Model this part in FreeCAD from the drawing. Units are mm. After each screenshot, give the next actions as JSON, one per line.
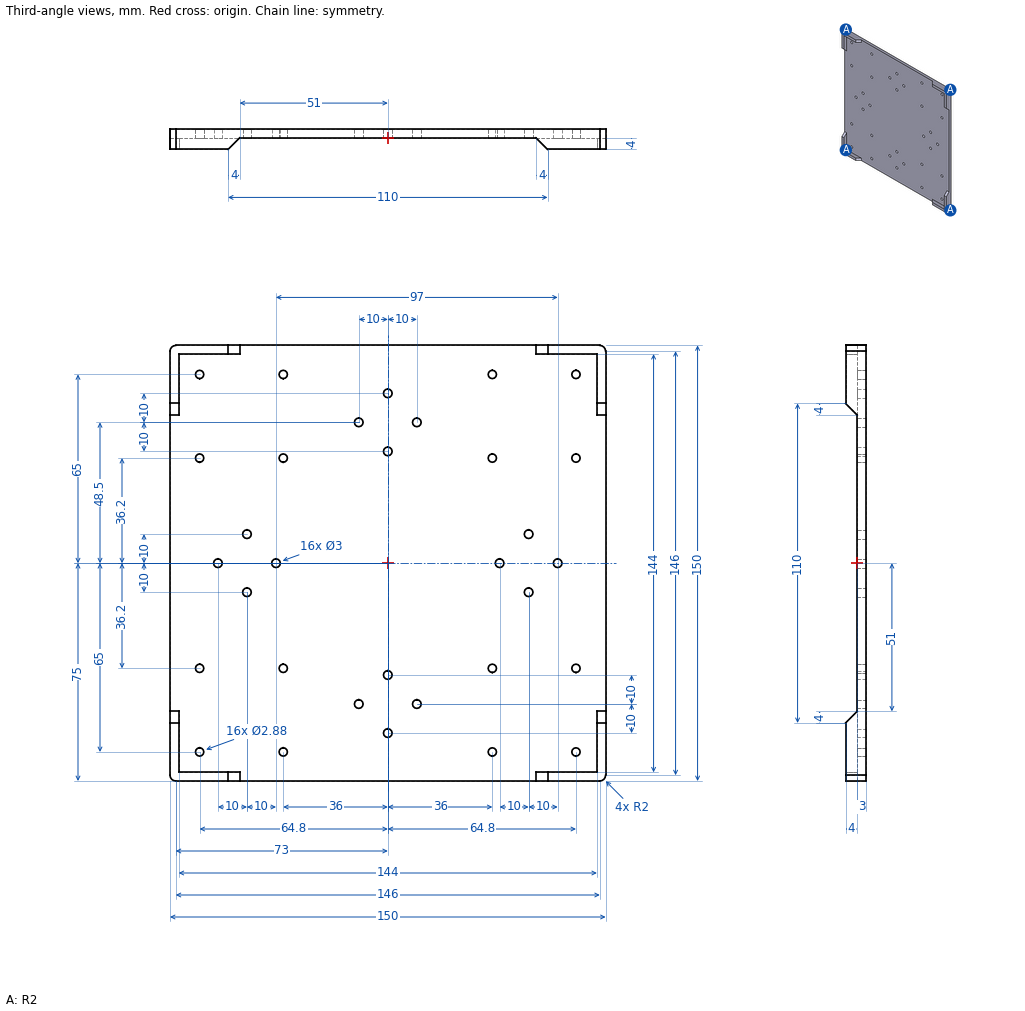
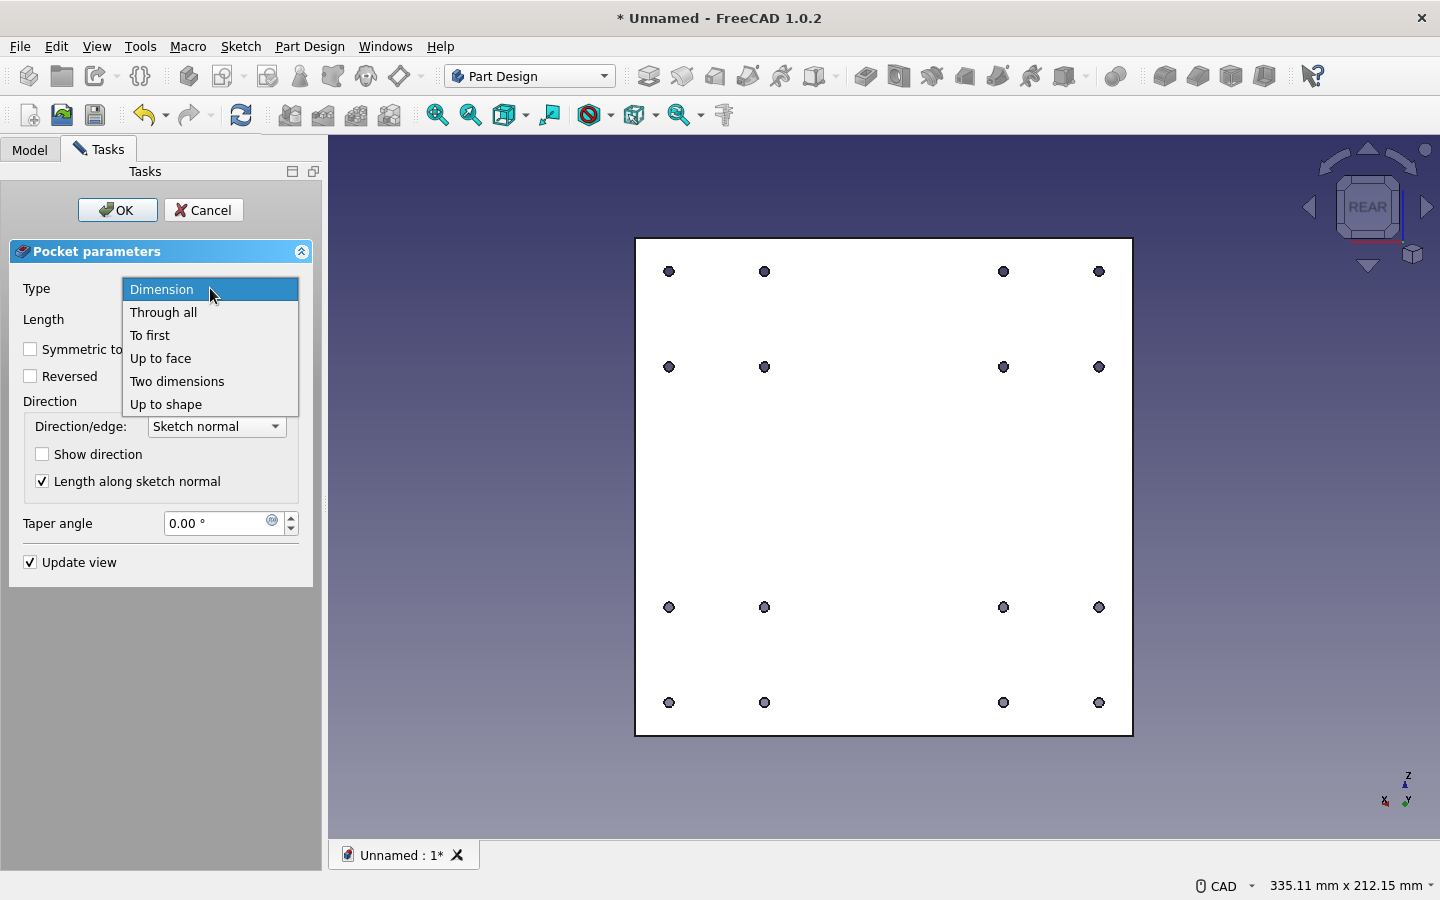
{"action": "left_click", "coordinate": [208, 312]}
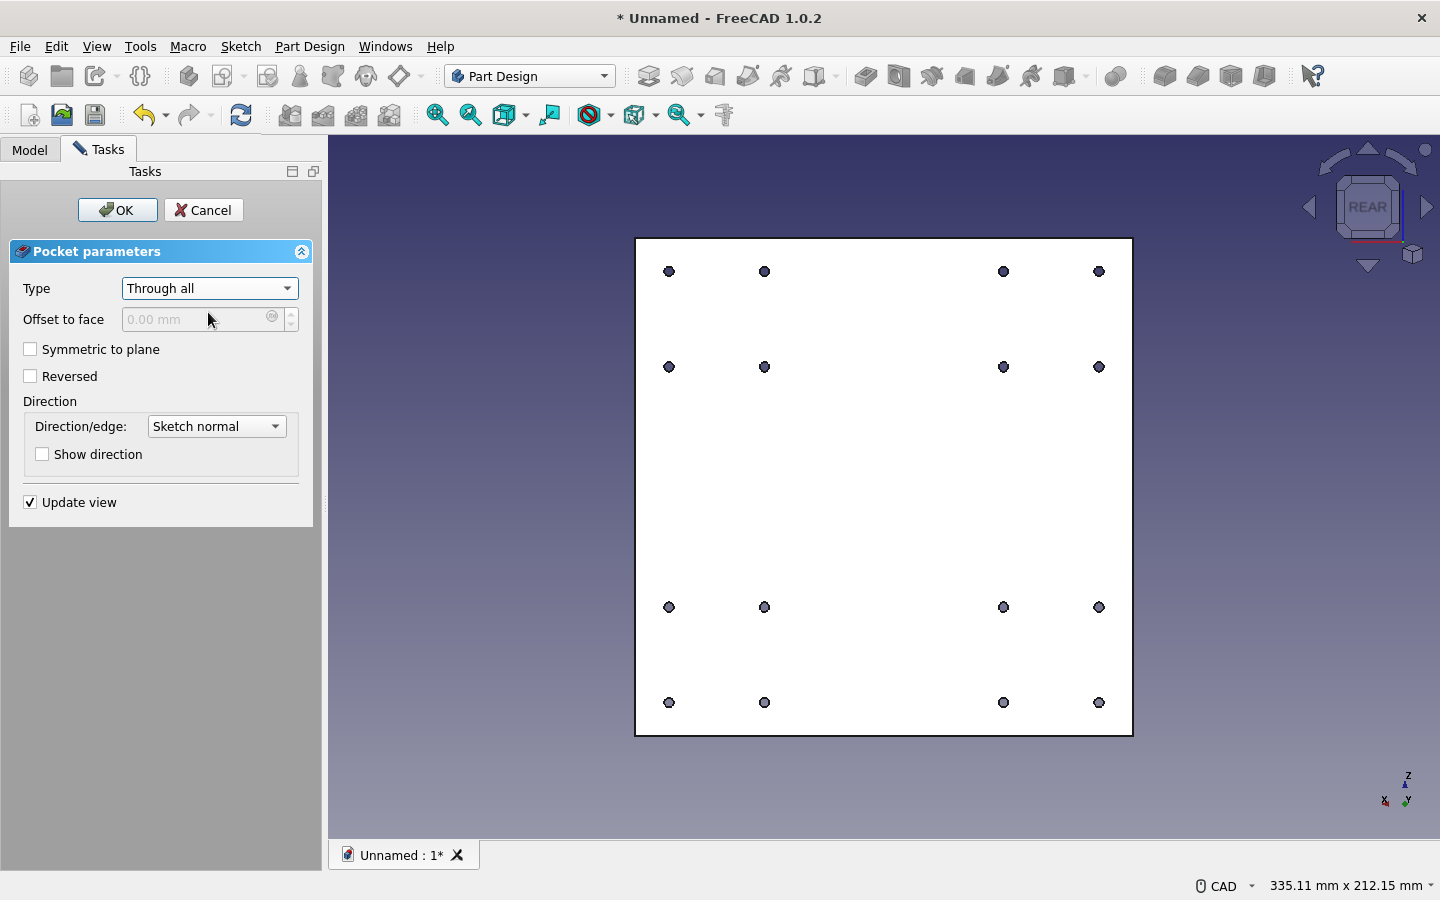
{"action": "left_click", "coordinate": [118, 210]}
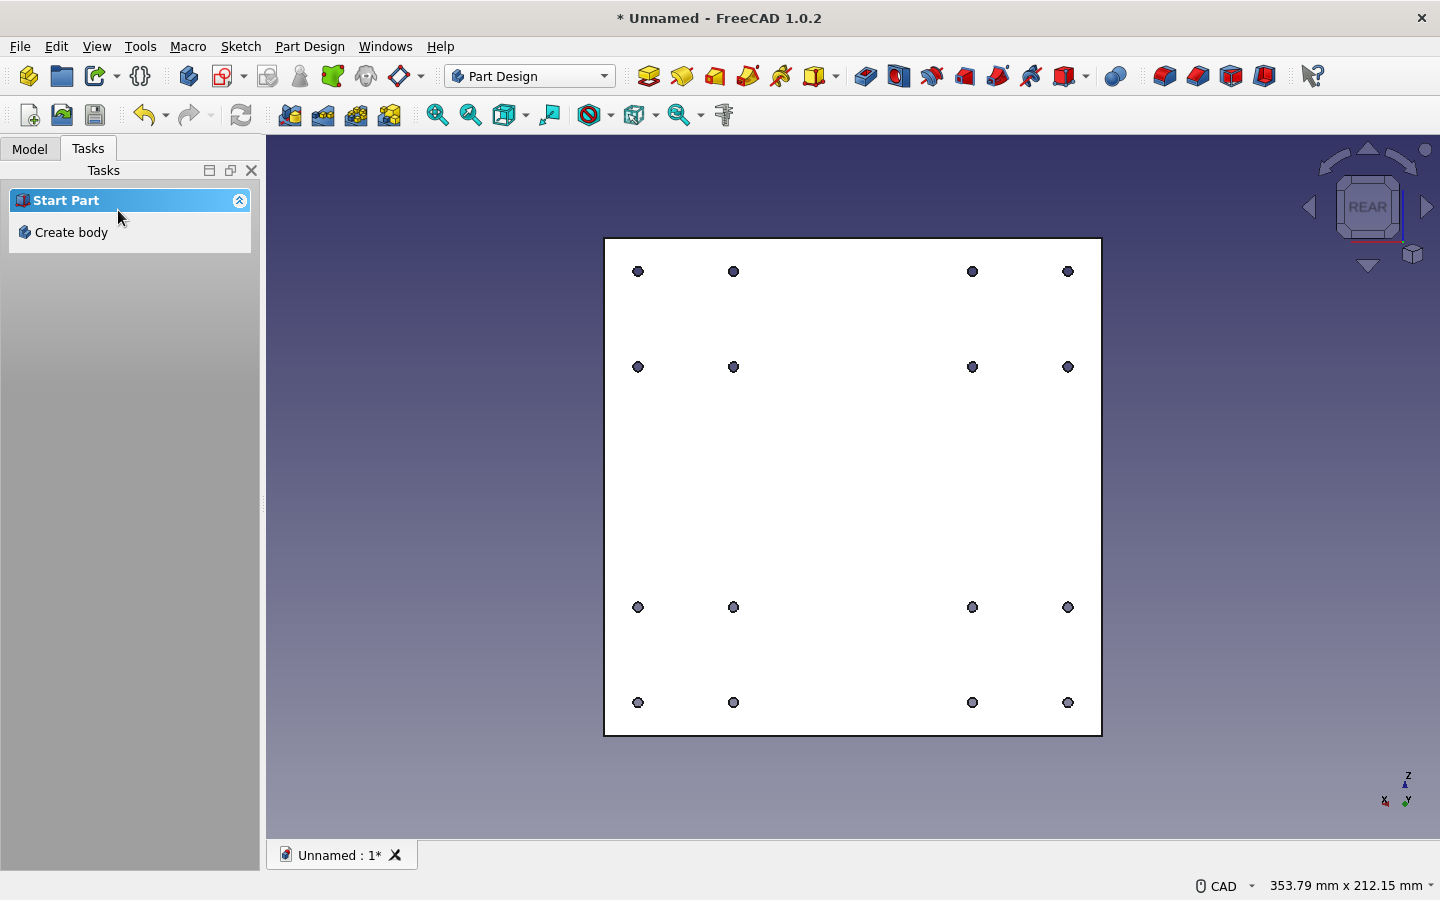
{"action": "left_click", "coordinate": [853, 486]}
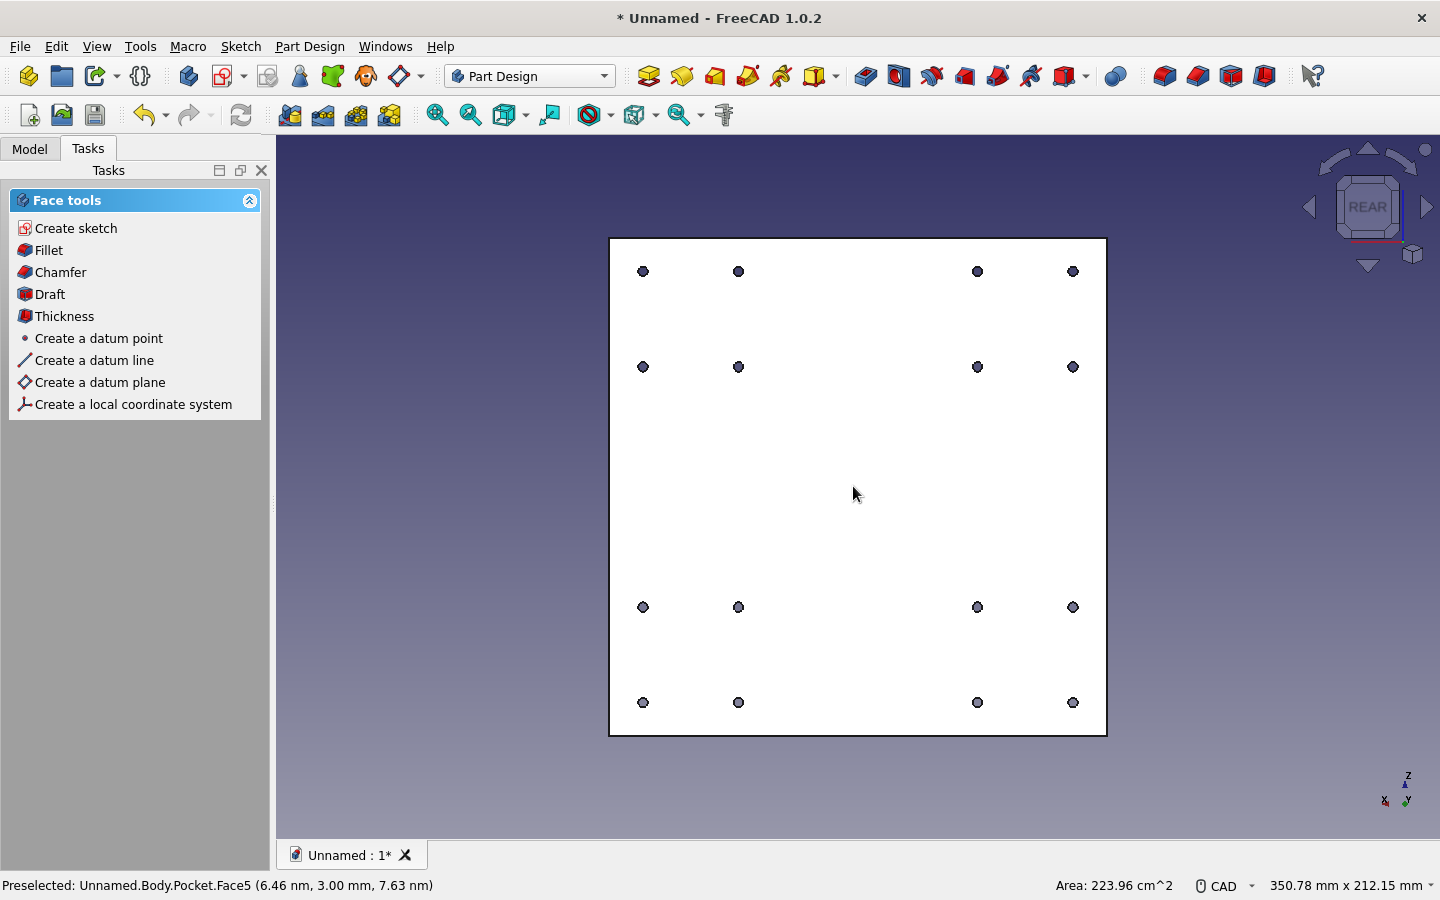
{"action": "left_click", "coordinate": [222, 76]}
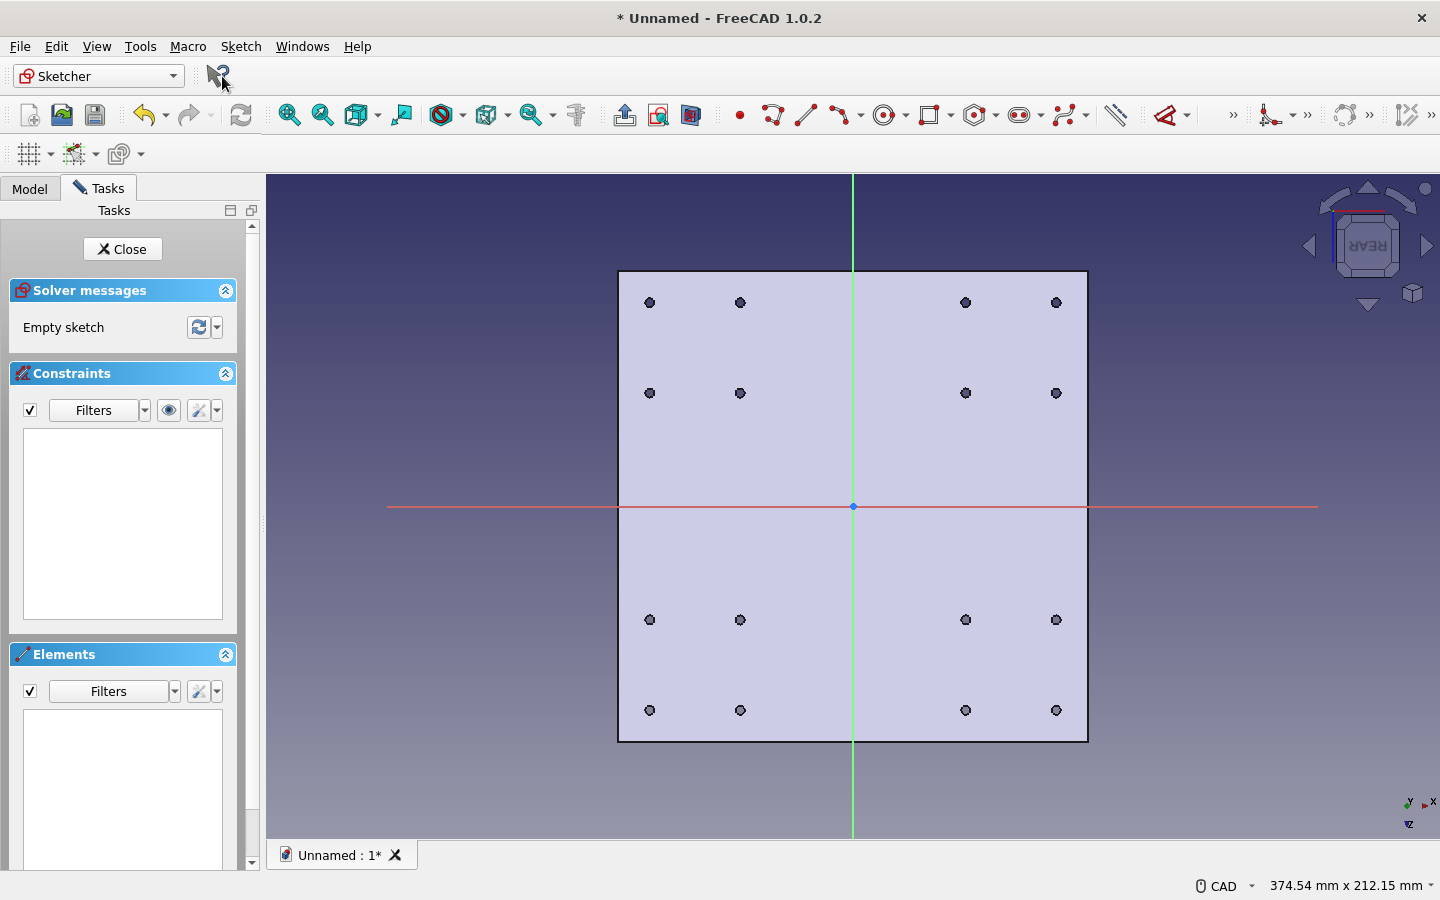
{"action": "left_click", "coordinate": [884, 116]}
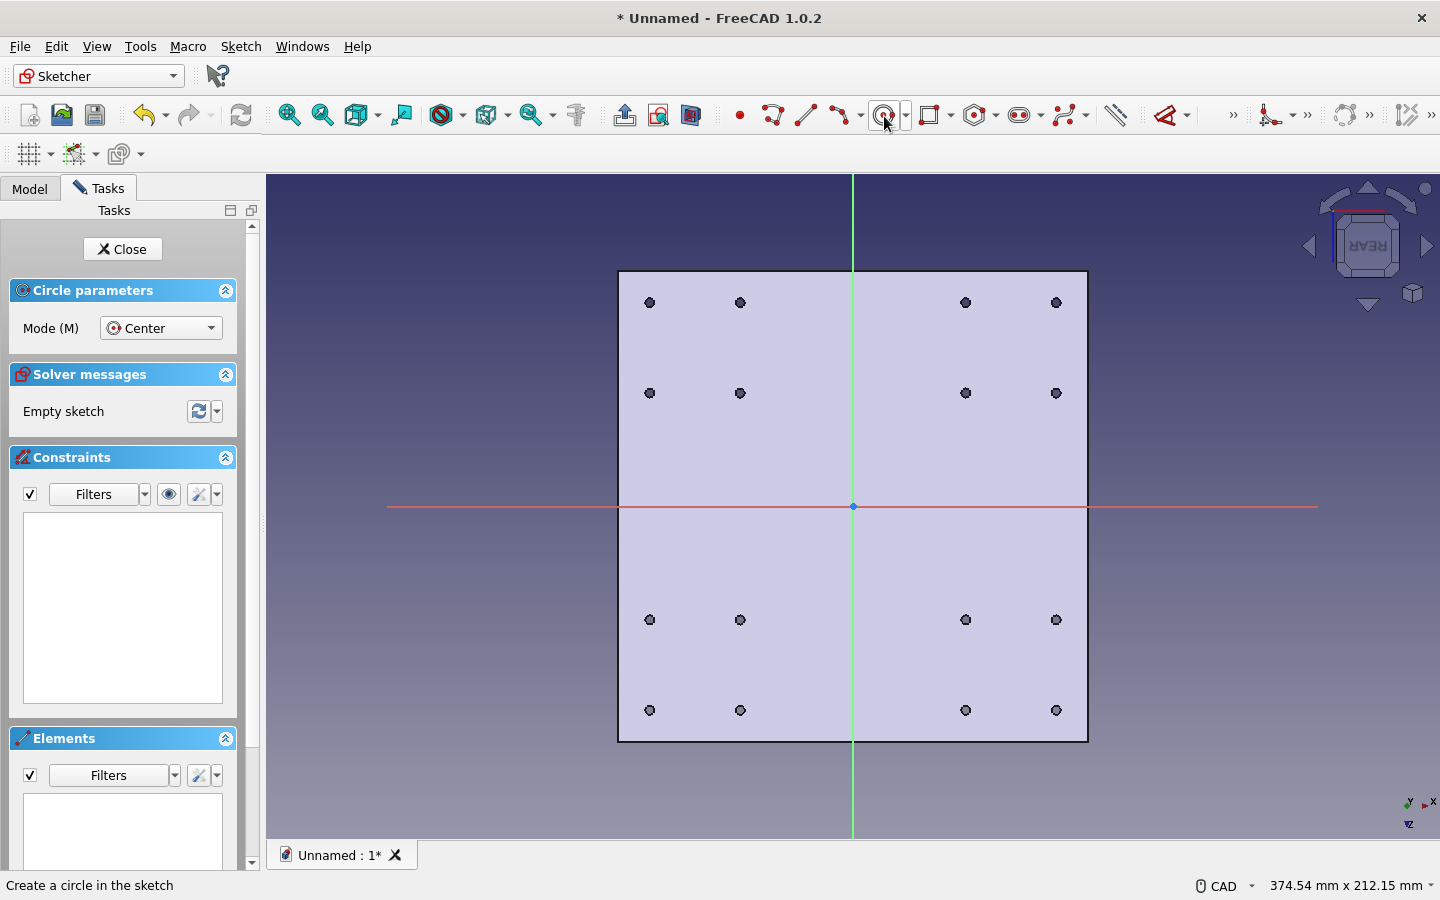
{"action": "scroll", "coordinate": [732, 506], "scroll_direction": "up", "scroll_amount": 8}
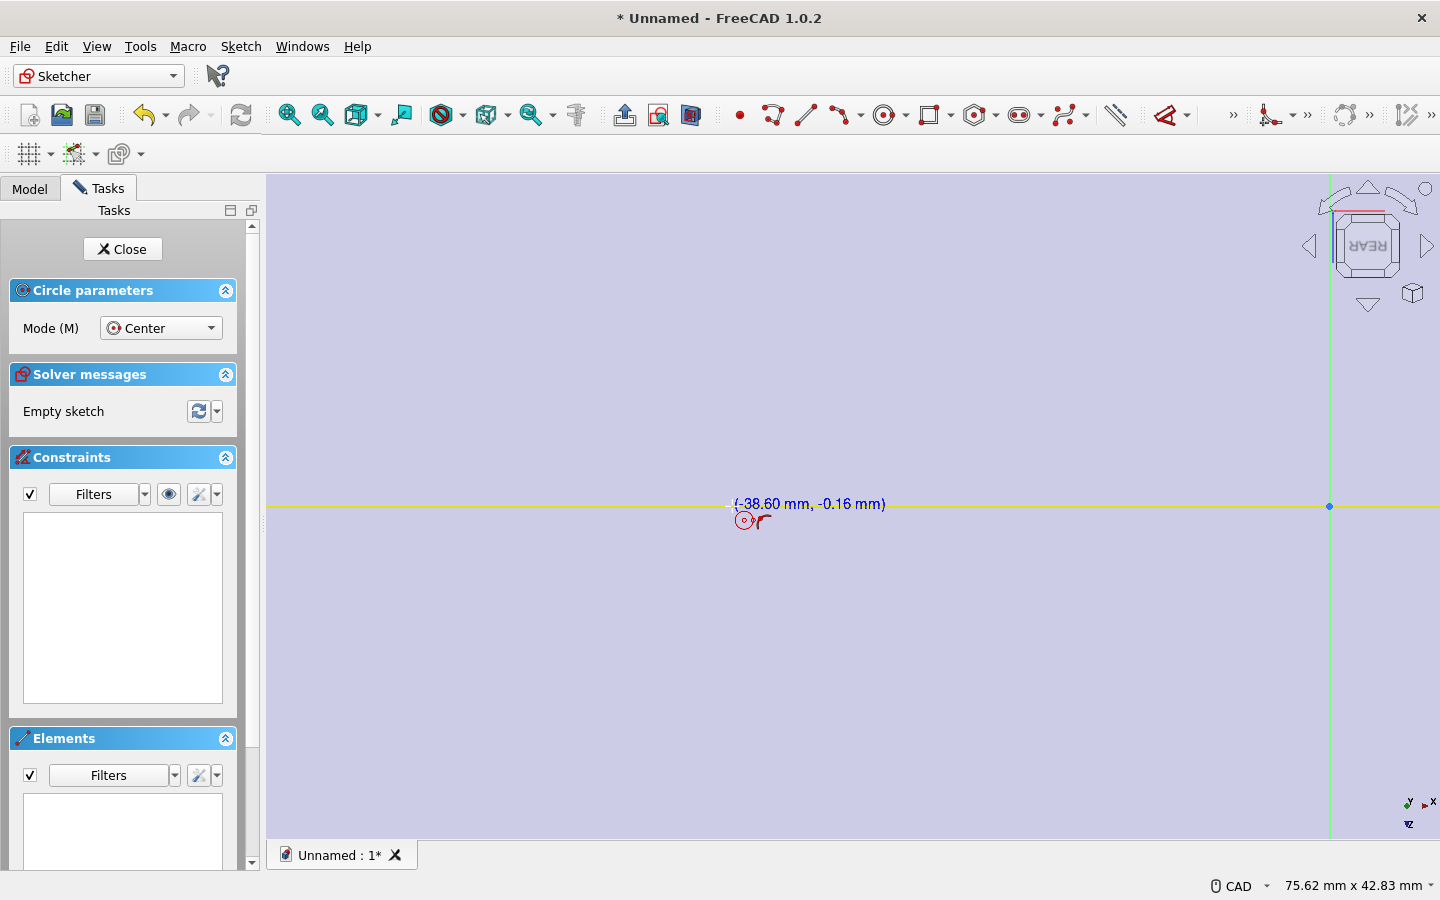
{"action": "scroll", "coordinate": [606, 507], "scroll_direction": "down", "scroll_amount": 7}